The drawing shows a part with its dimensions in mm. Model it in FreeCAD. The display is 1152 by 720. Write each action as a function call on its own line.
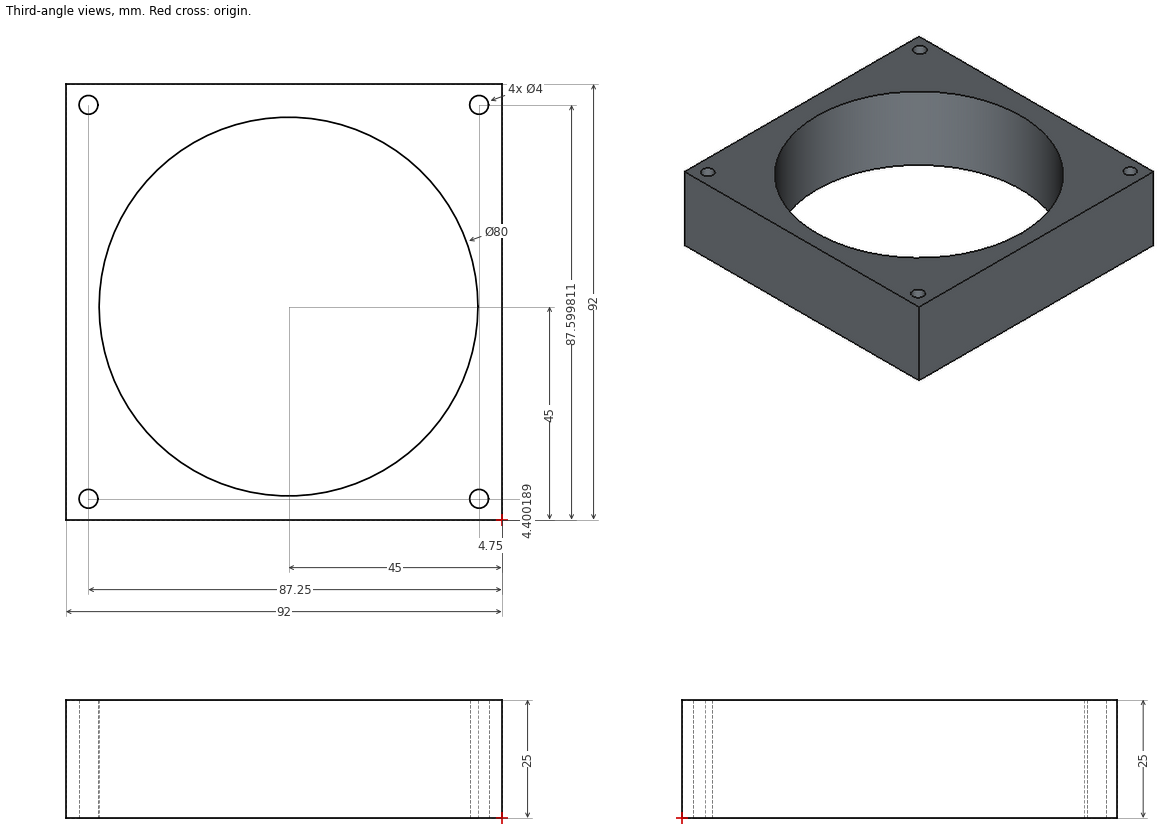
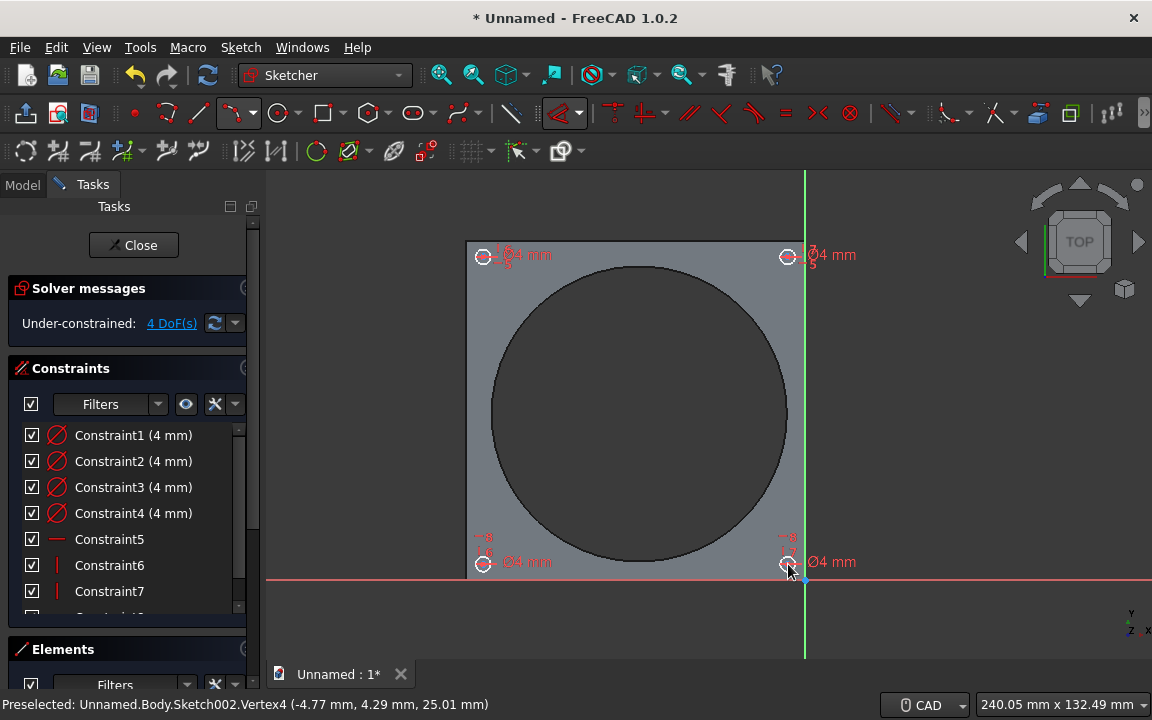
scroll(788, 257, up, 5)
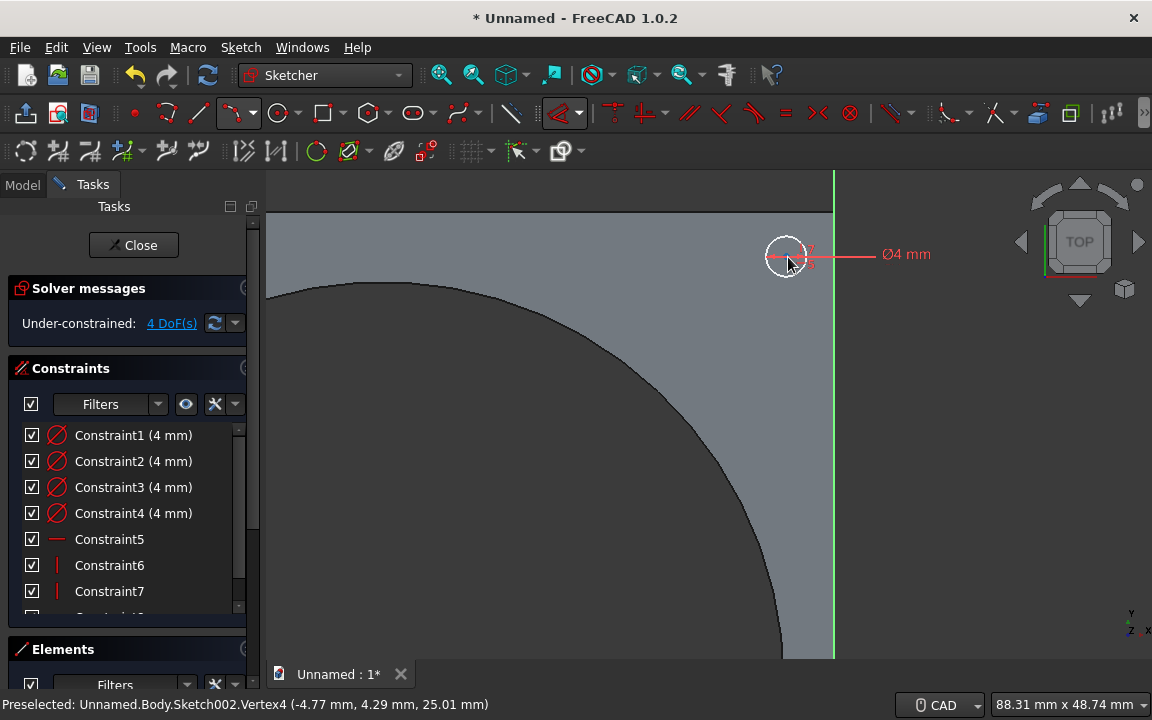
click(786, 257)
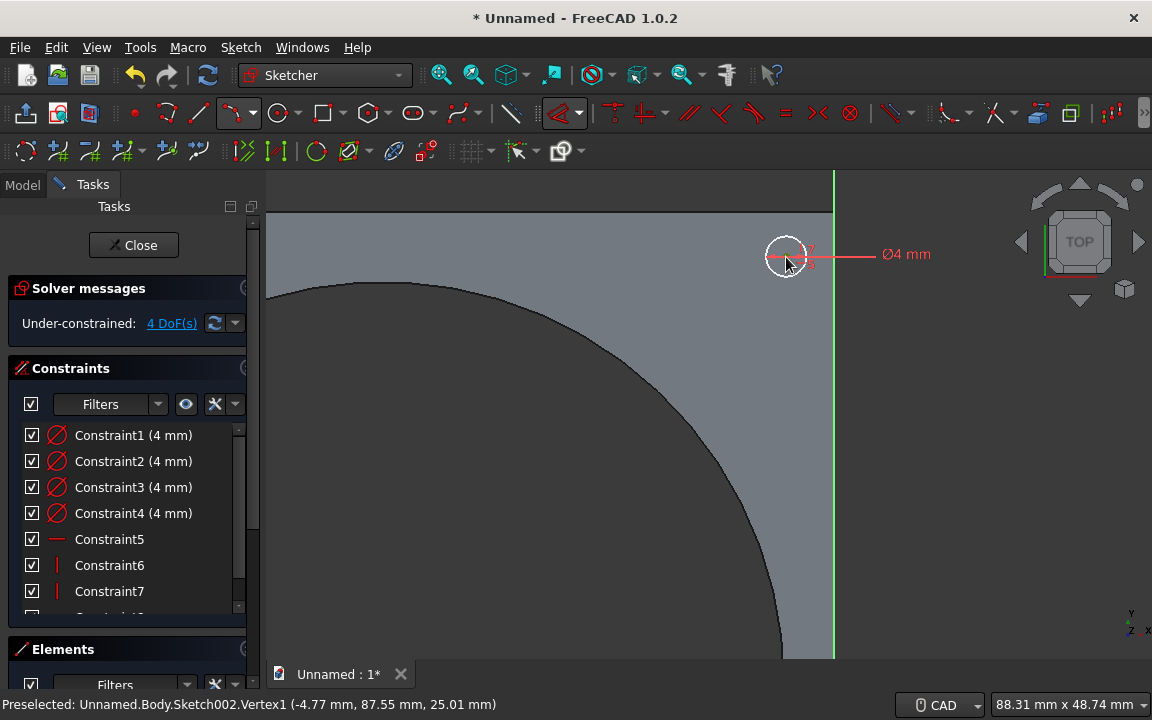
key(l)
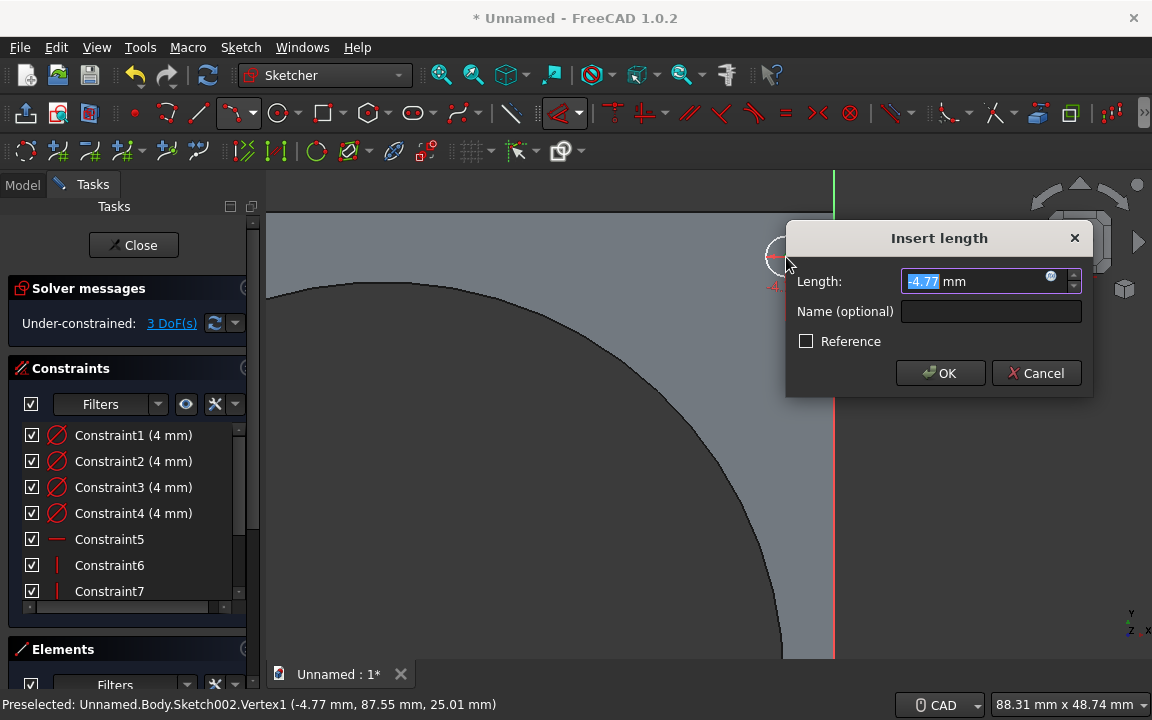
text(-4.75)
key(Return)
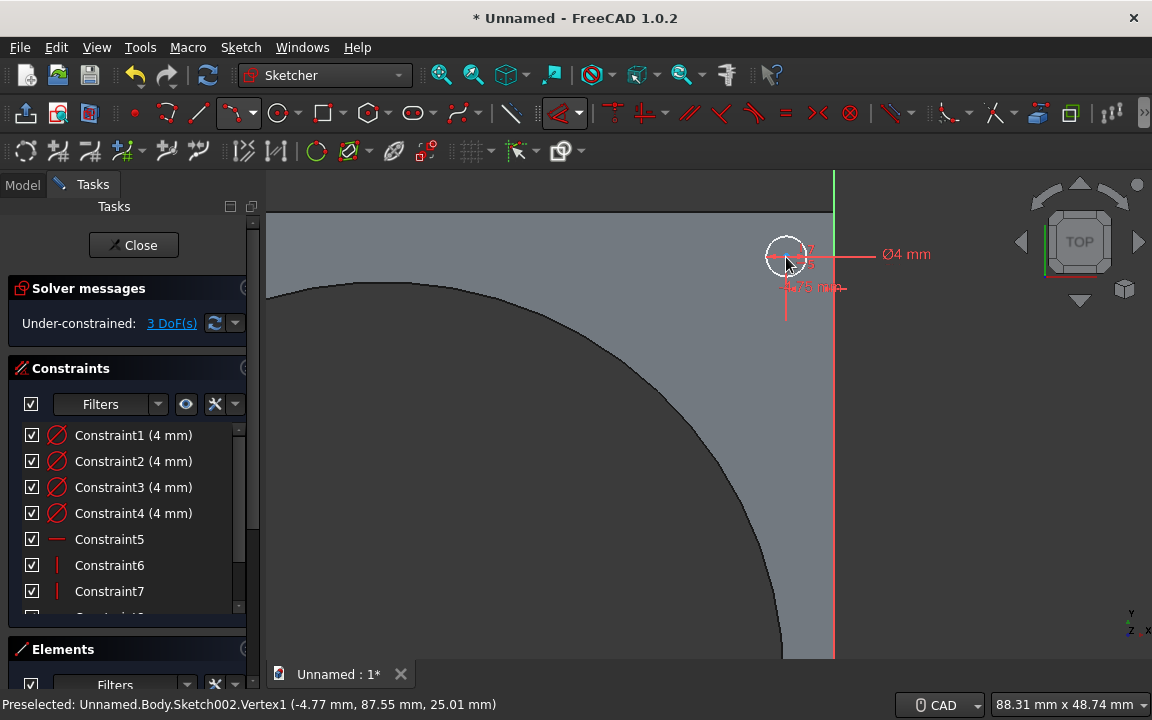
scroll(788, 257, down, 5)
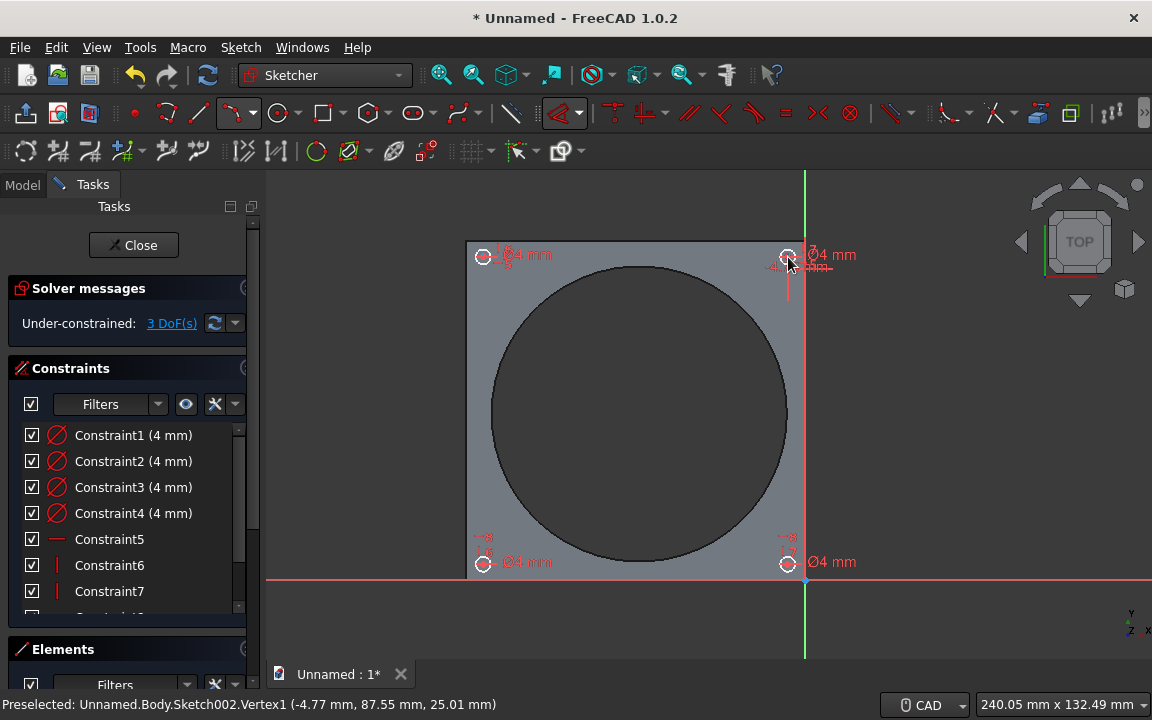
click(483, 257)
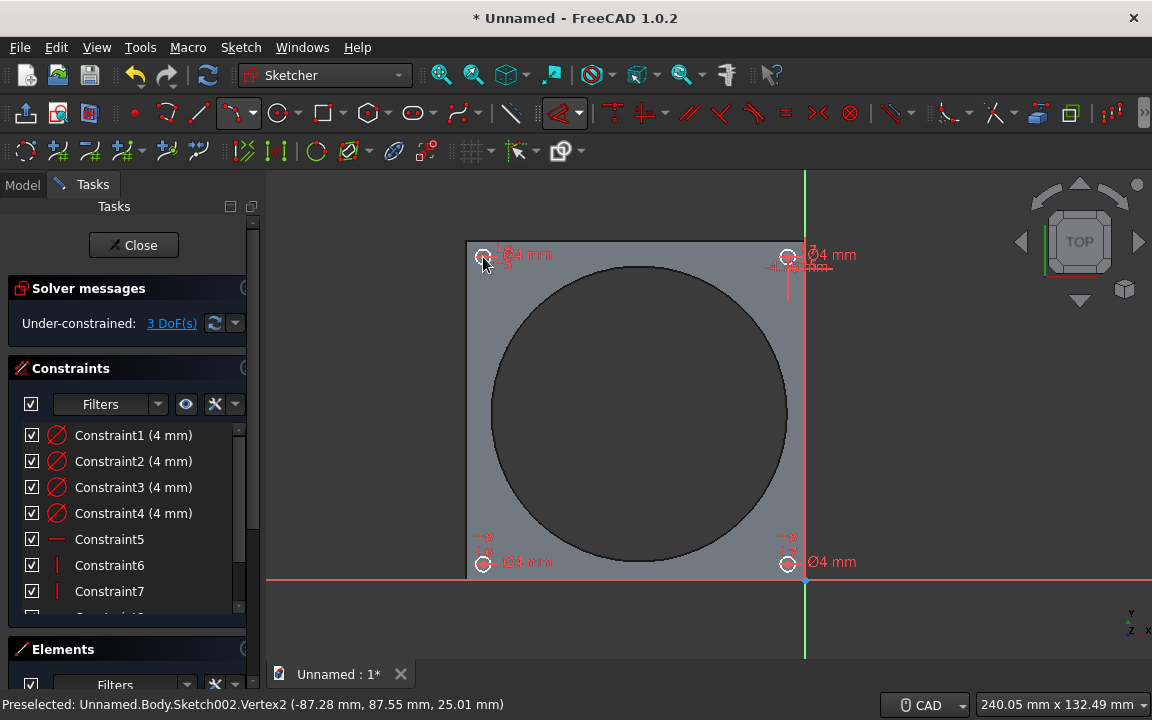
key(l)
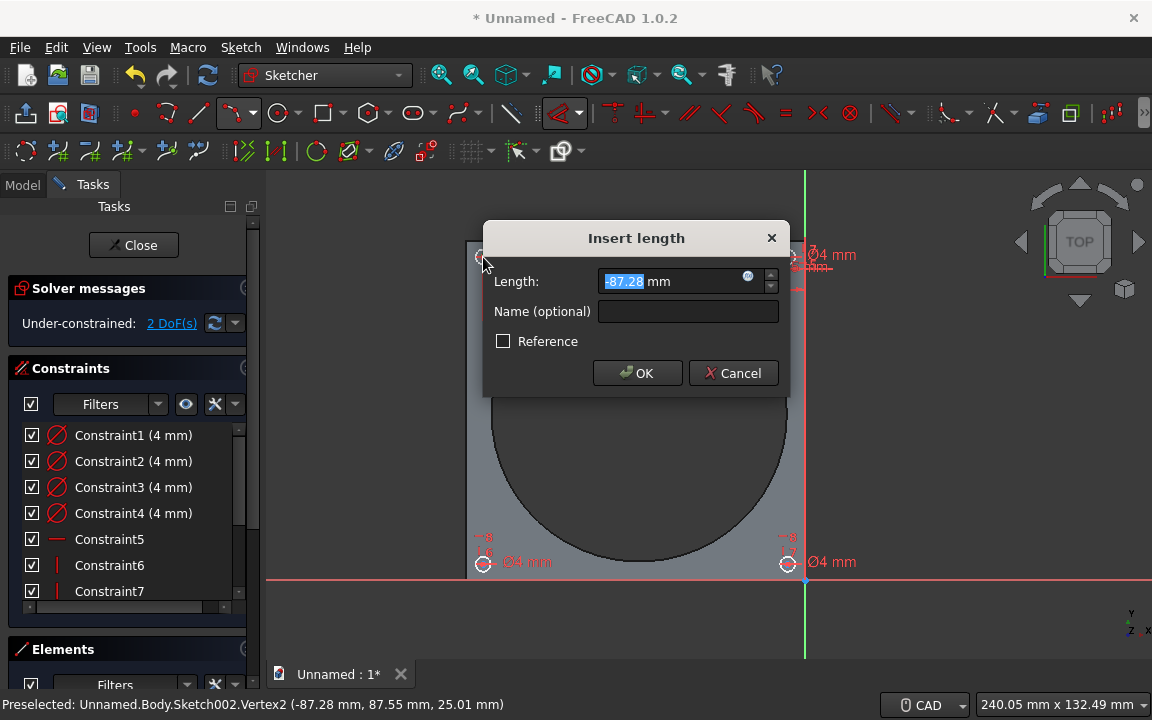
text(-87.25)
key(Return)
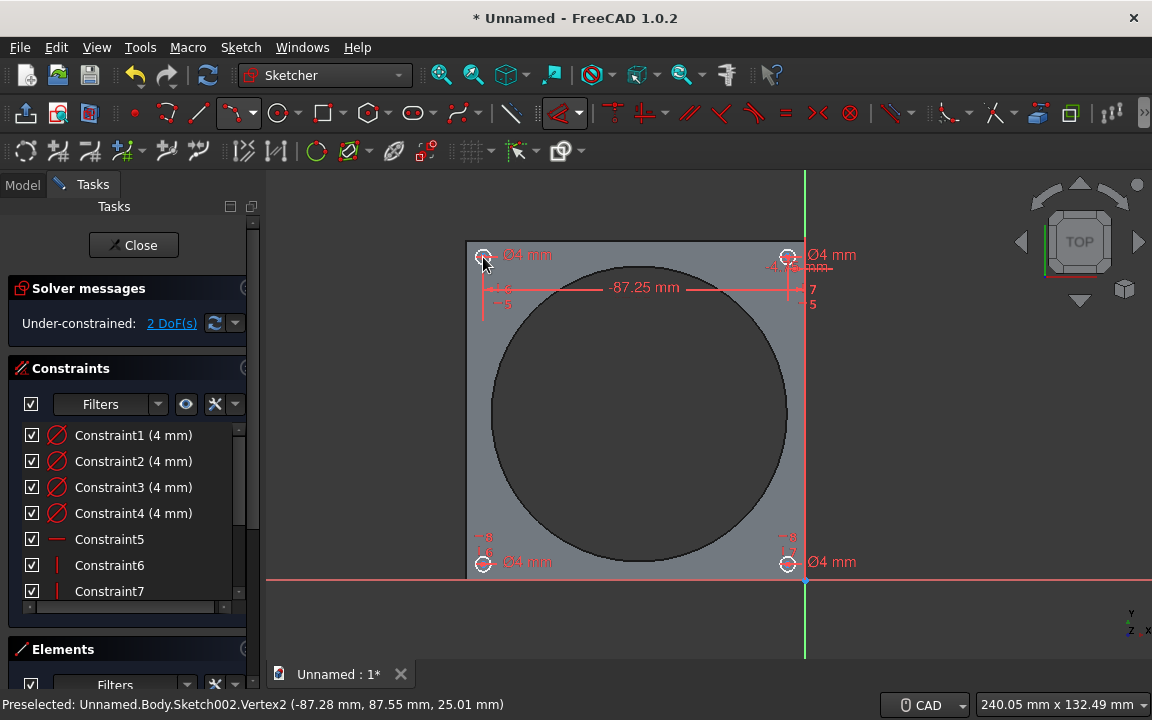
scroll(483, 564, up, 5)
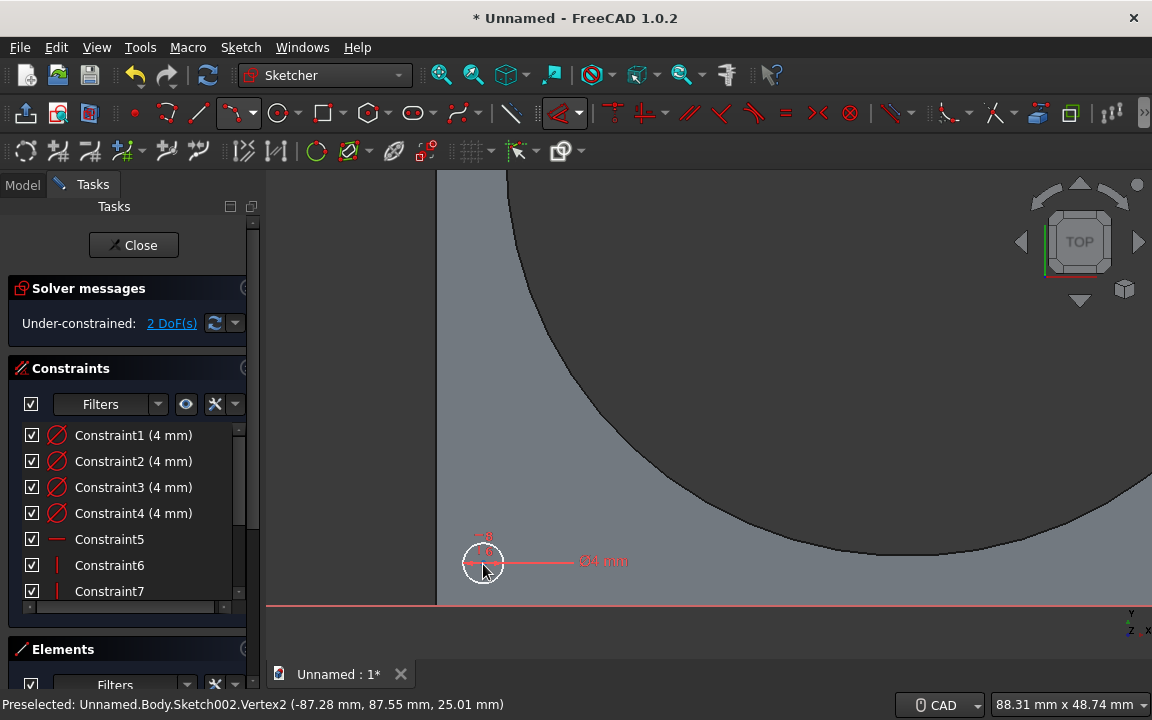
click(483, 563)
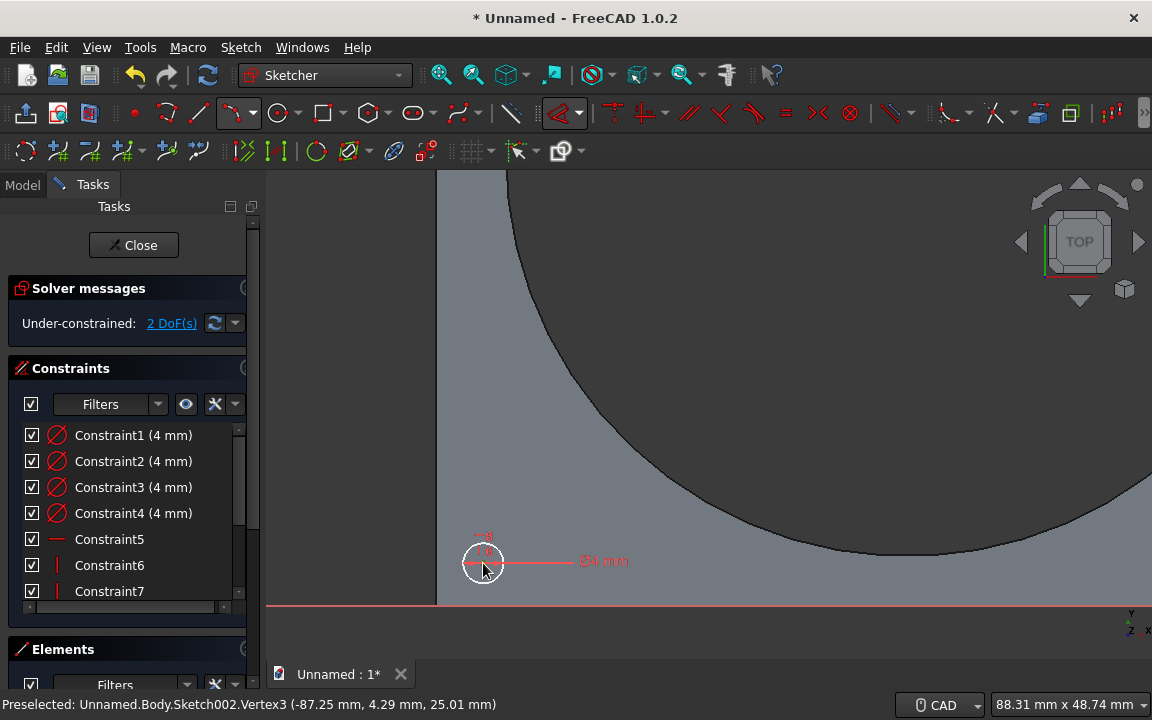
key(i)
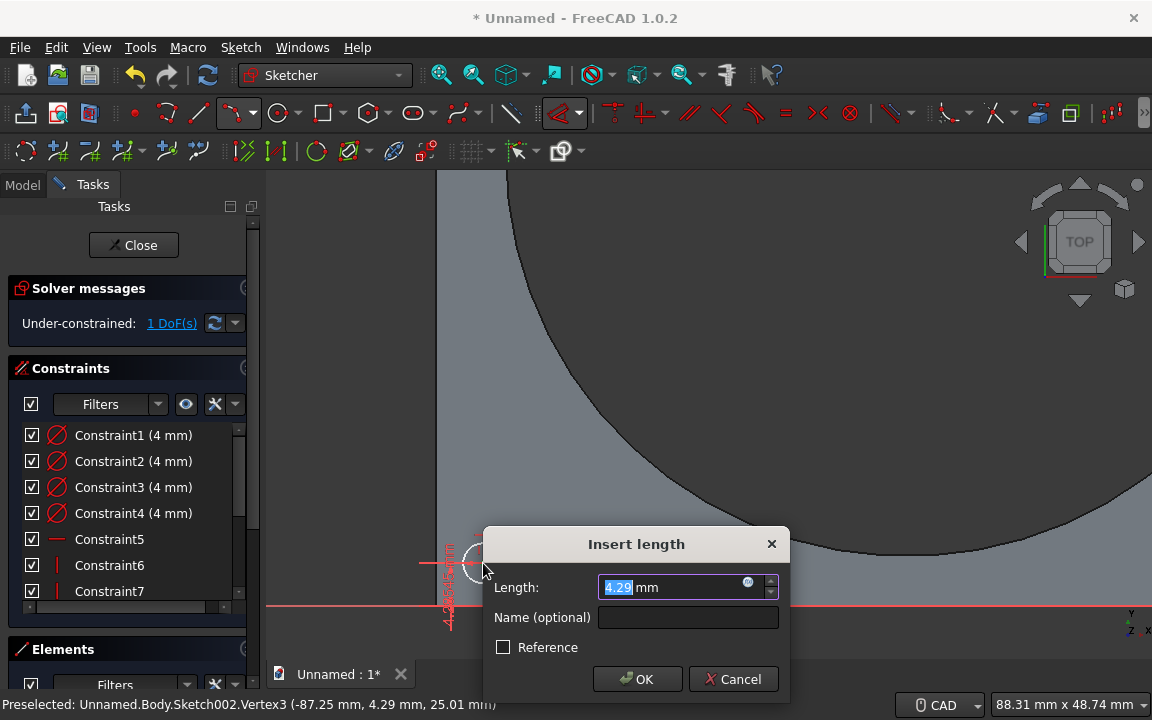
text(4.400189)
key(Return)